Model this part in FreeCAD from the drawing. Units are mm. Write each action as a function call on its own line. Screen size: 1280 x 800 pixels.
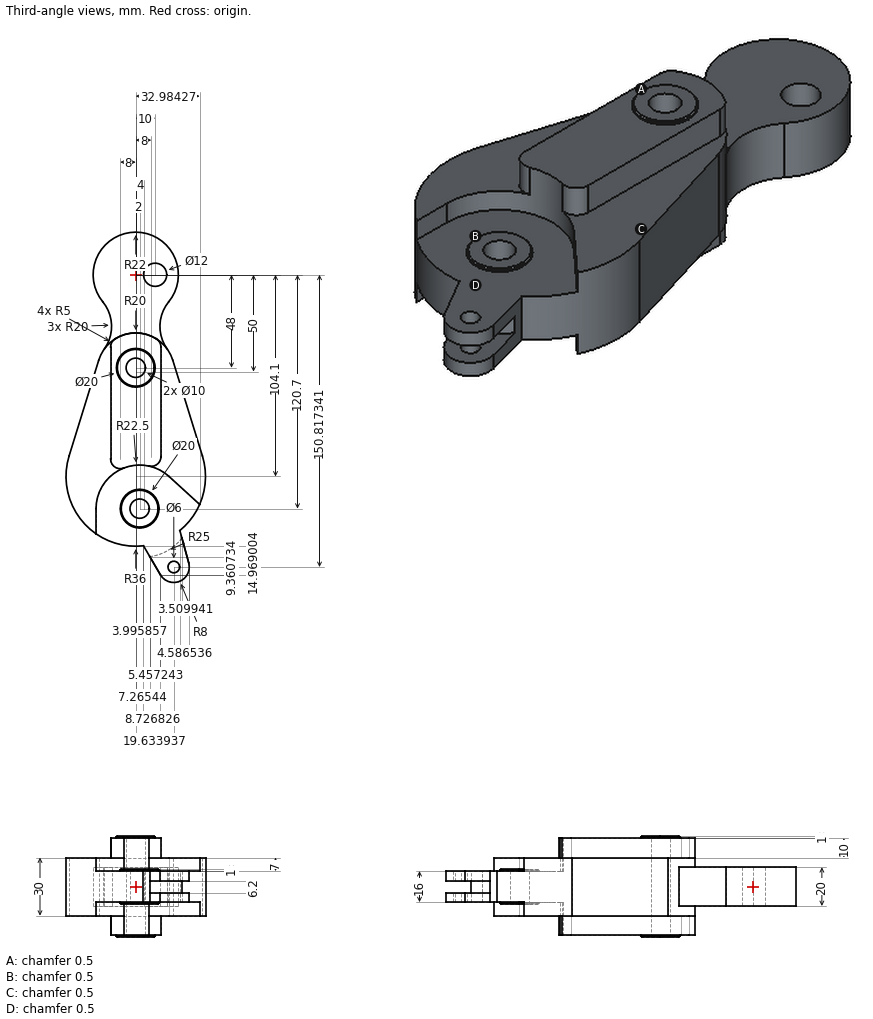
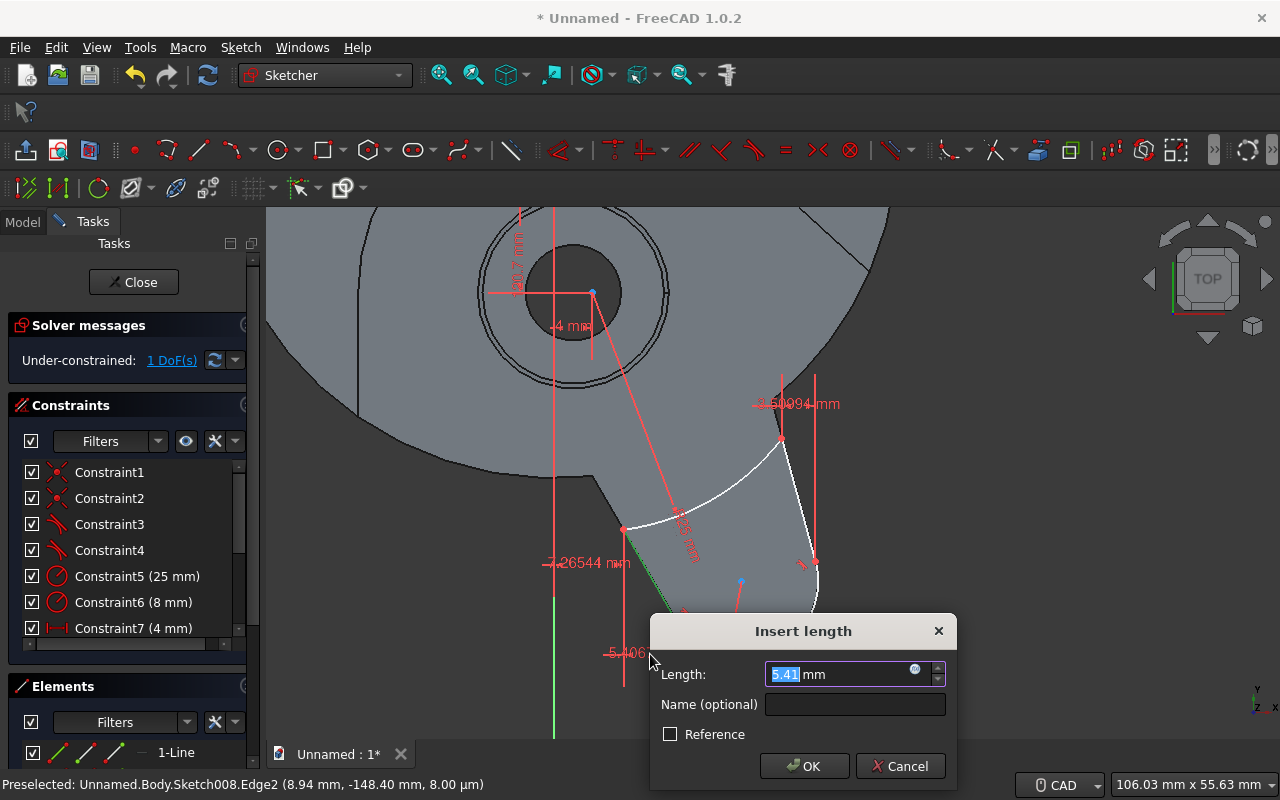
text(5.457243)
key(Return)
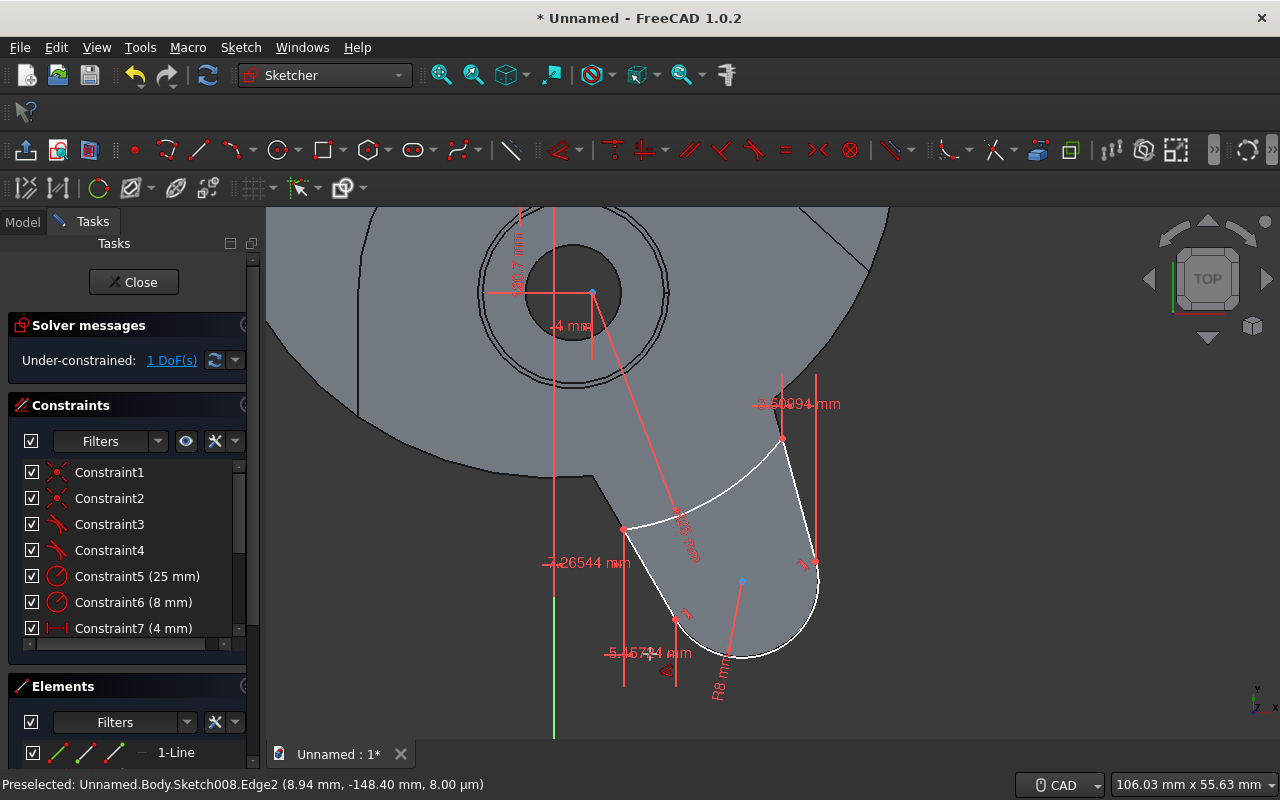
click(639, 557)
click(590, 595)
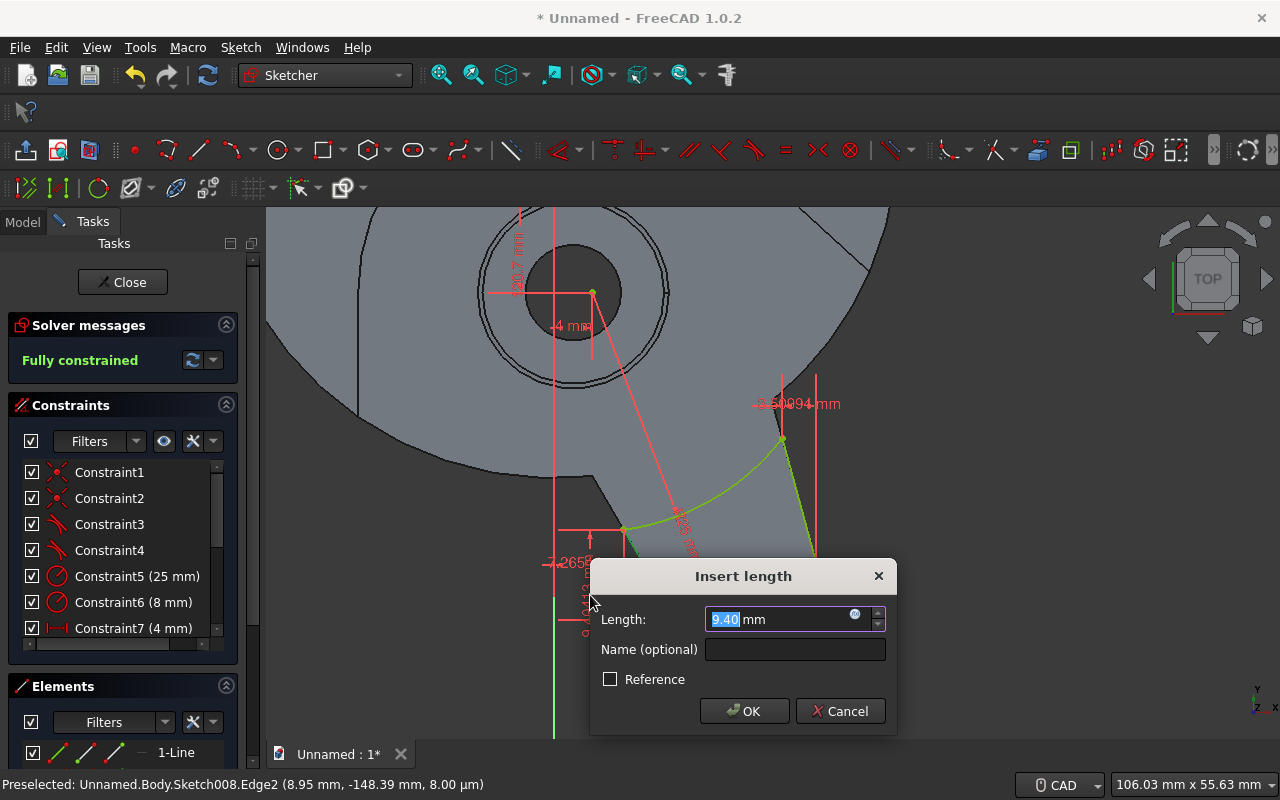
text(9.360734)
key(Return)
key(Escape)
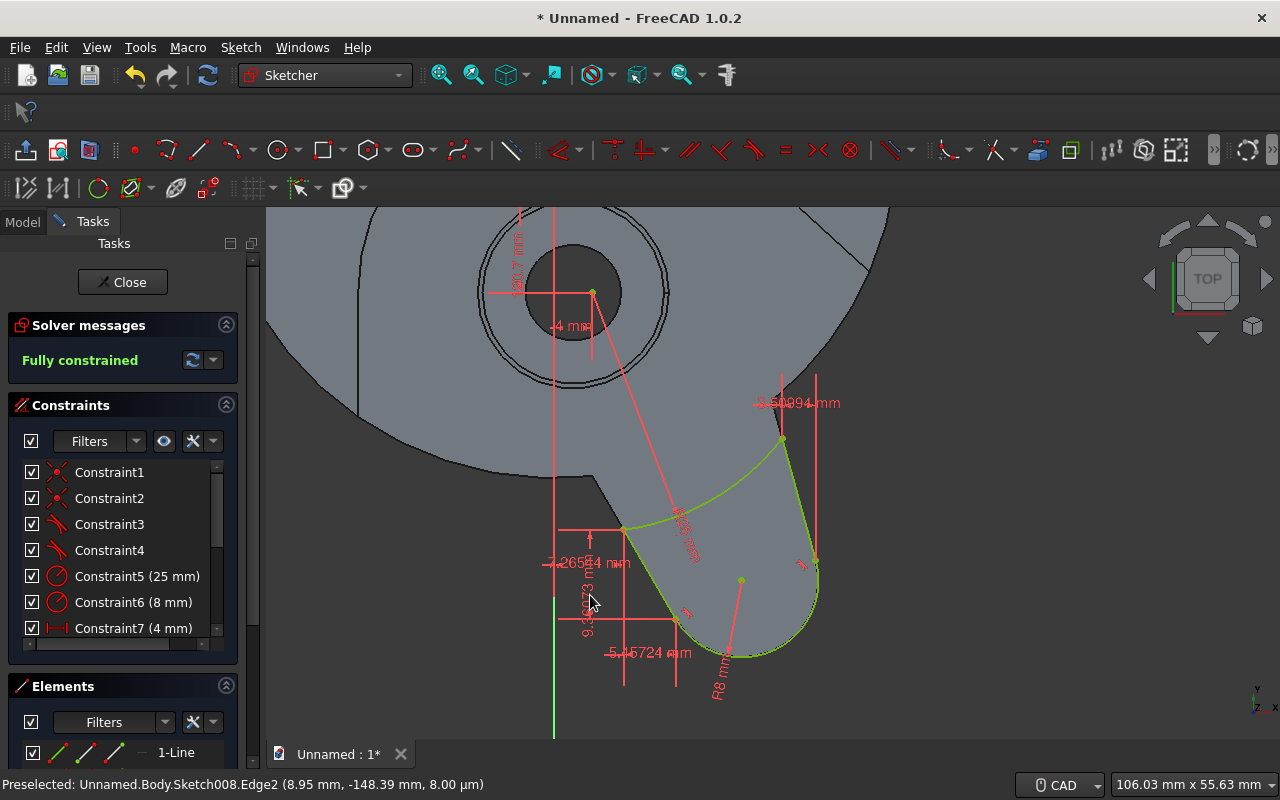
click(123, 282)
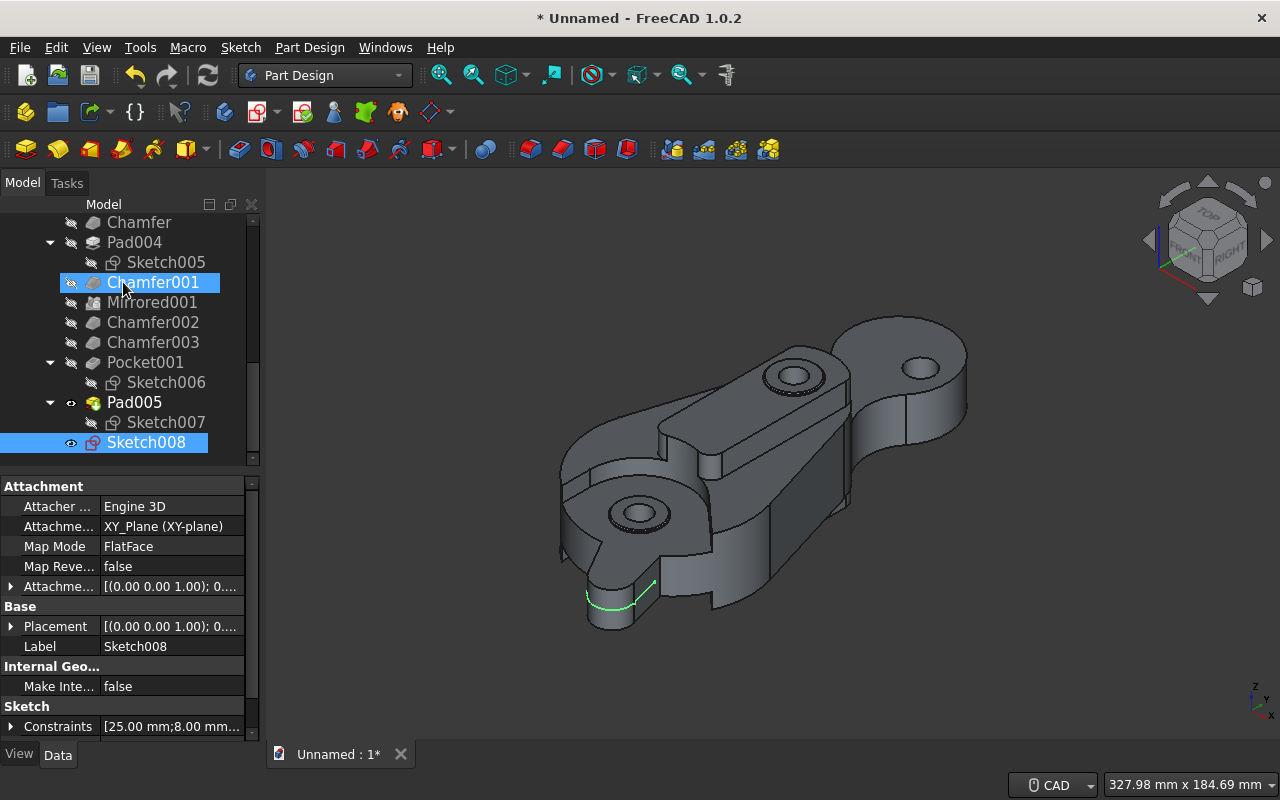
click(240, 150)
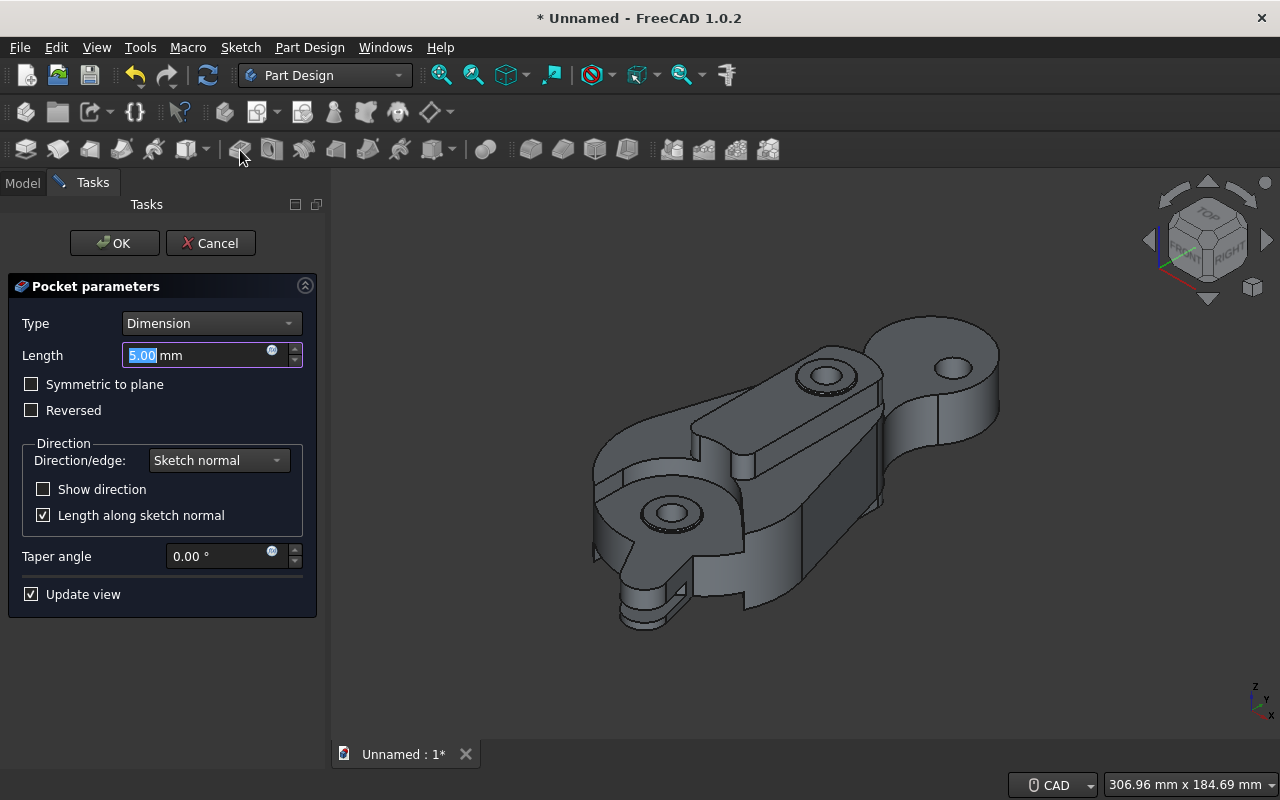
text(6.2)
key(Tab)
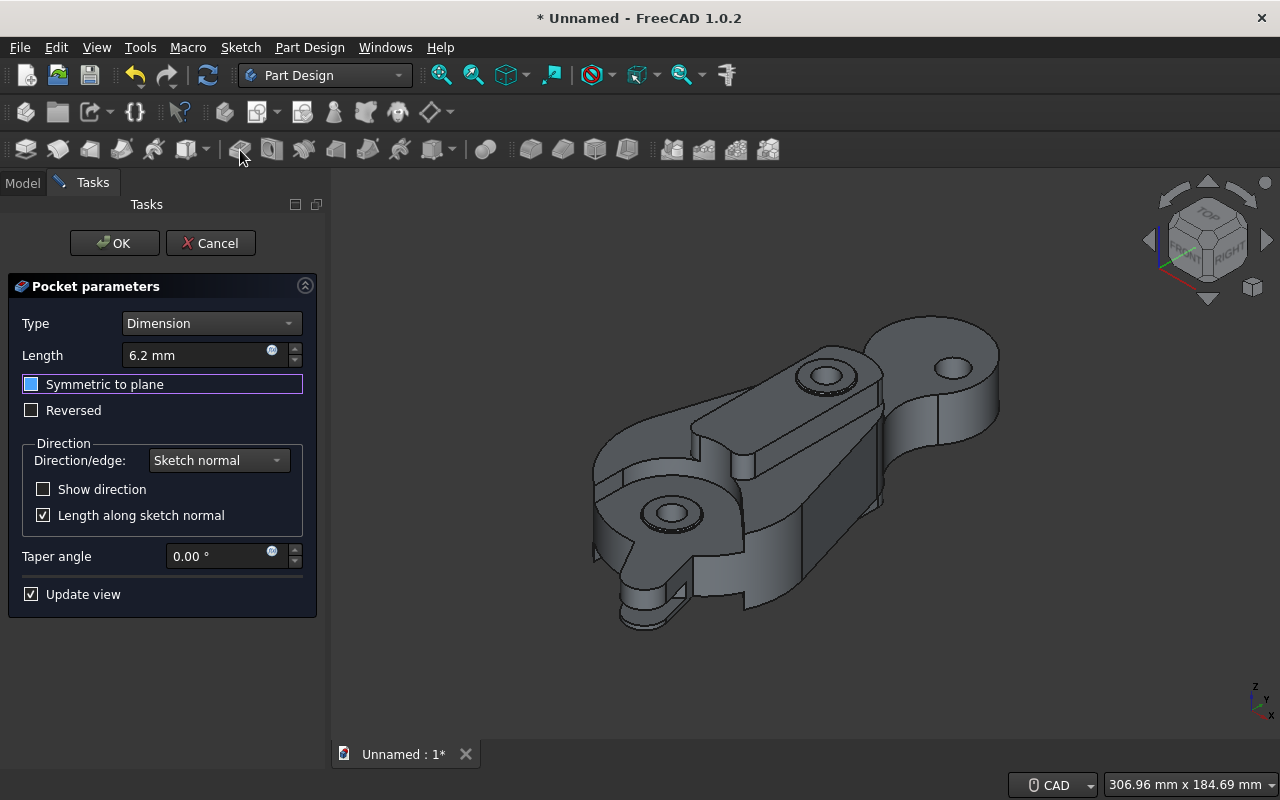
click(30, 384)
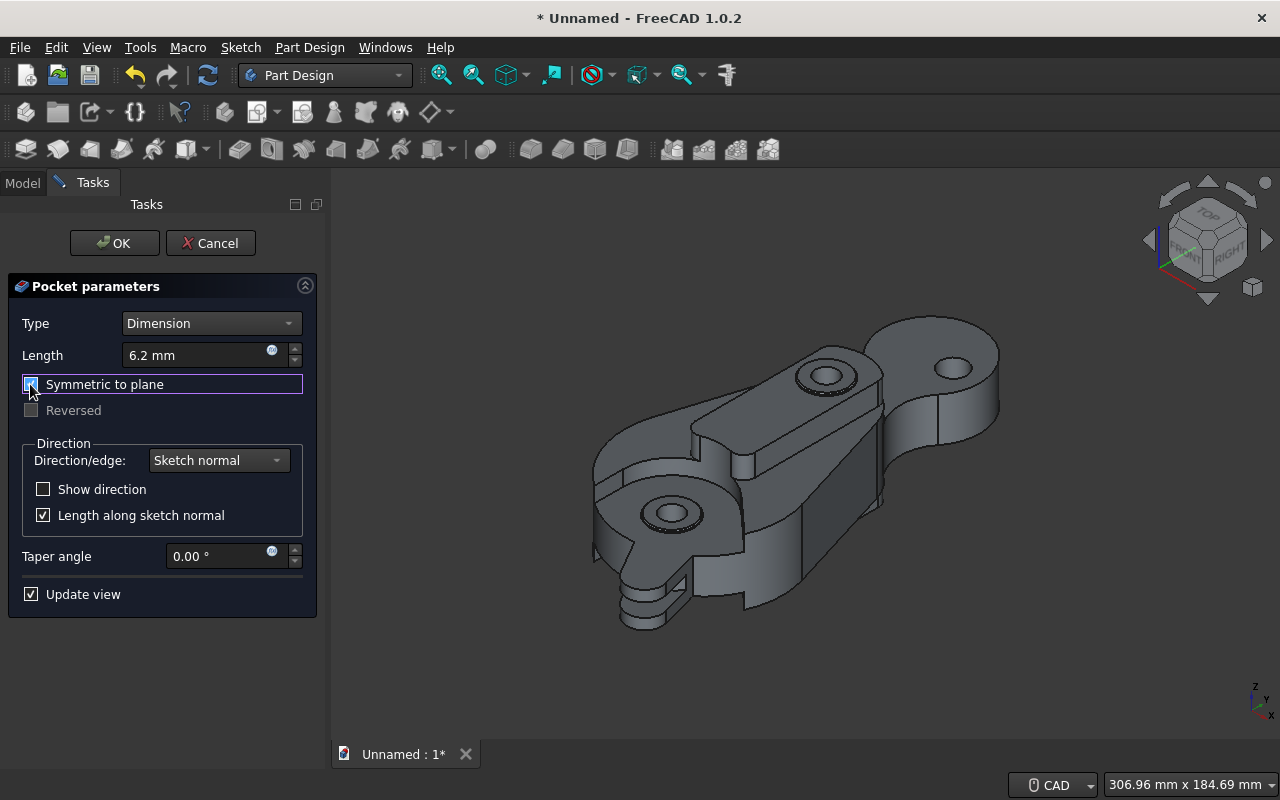
click(115, 243)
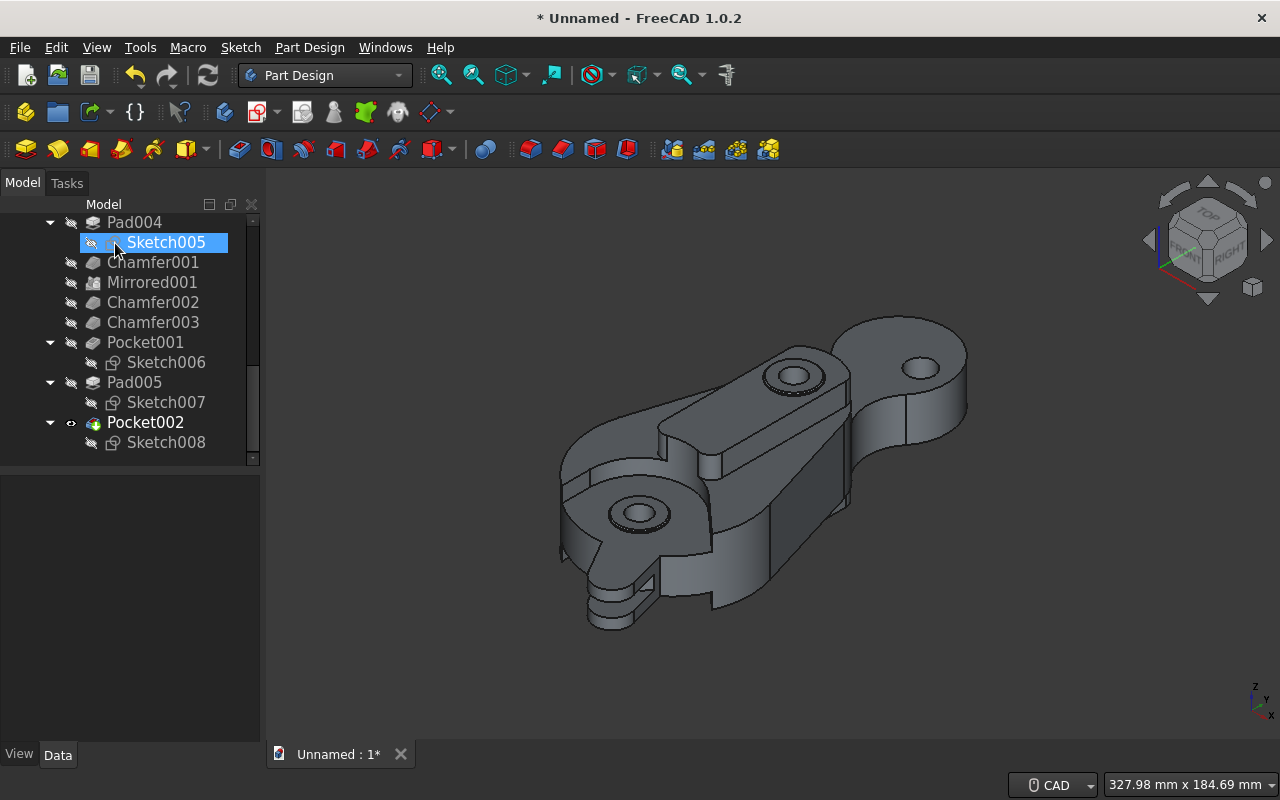
click(629, 550)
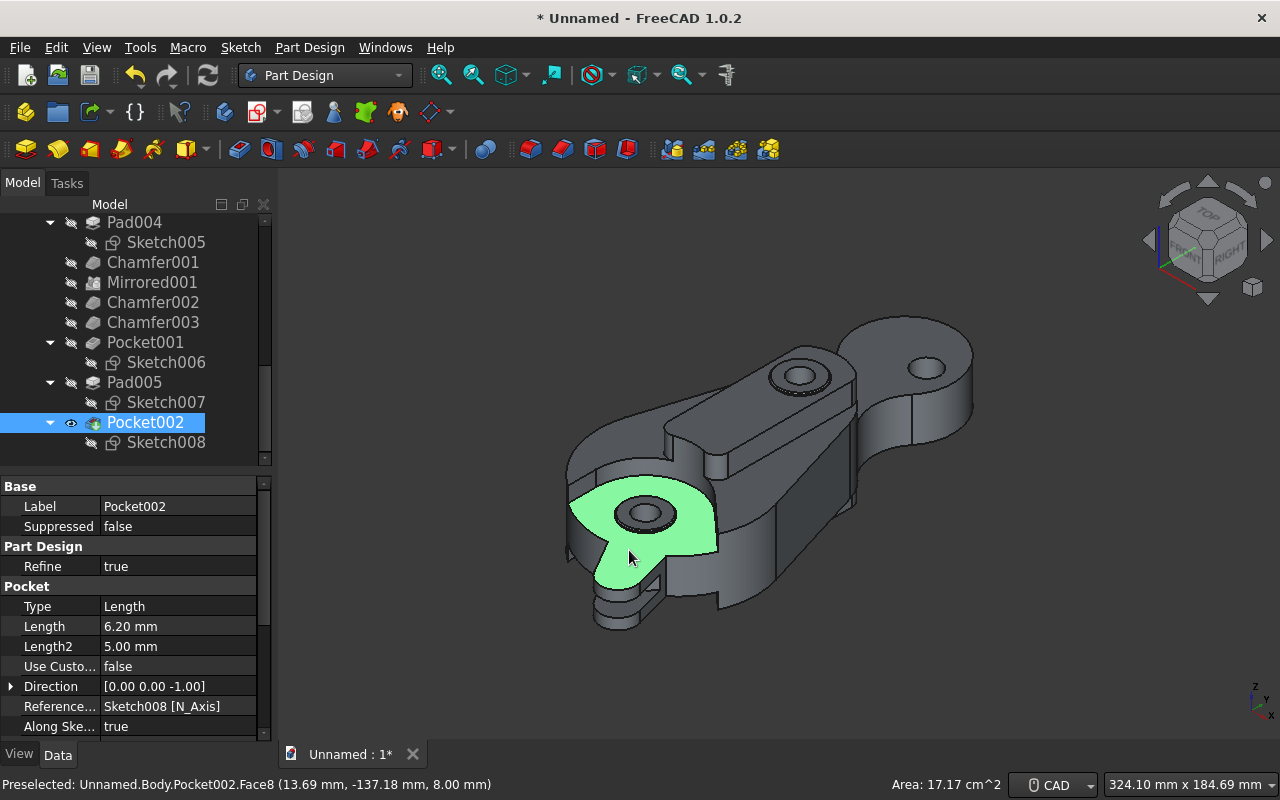
click(258, 112)